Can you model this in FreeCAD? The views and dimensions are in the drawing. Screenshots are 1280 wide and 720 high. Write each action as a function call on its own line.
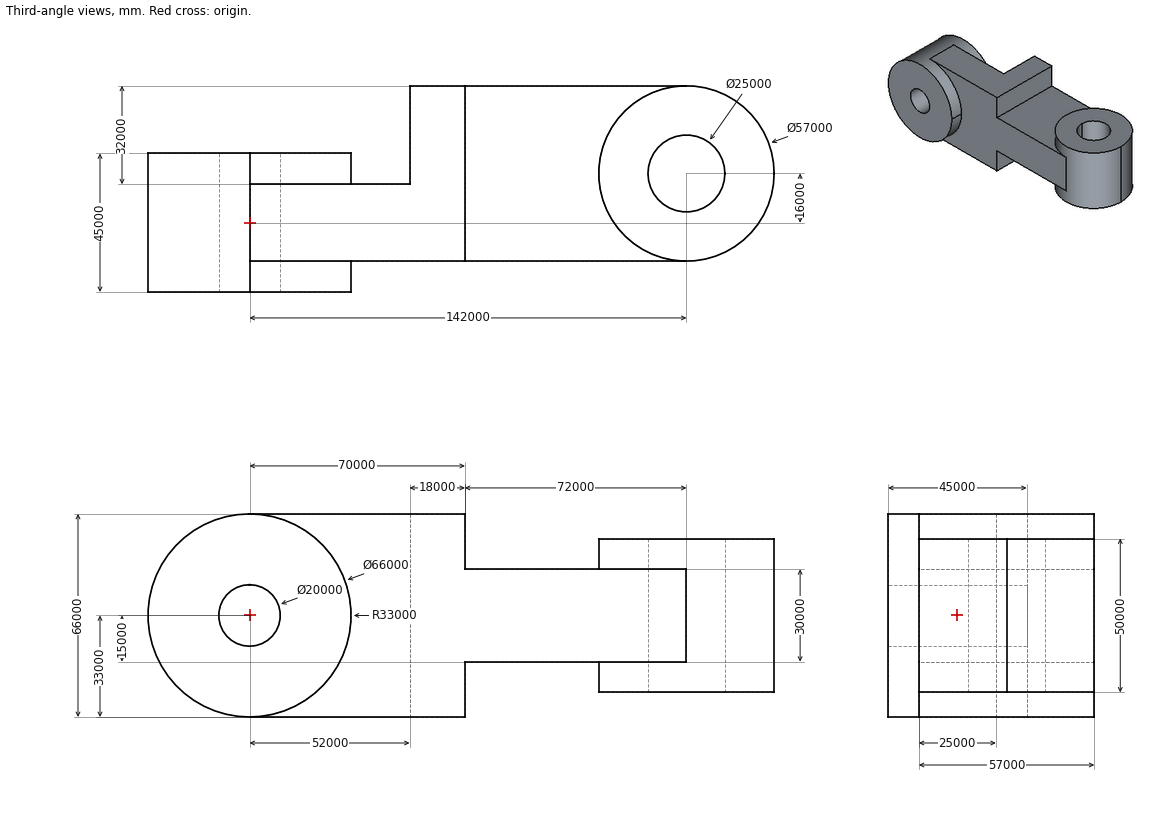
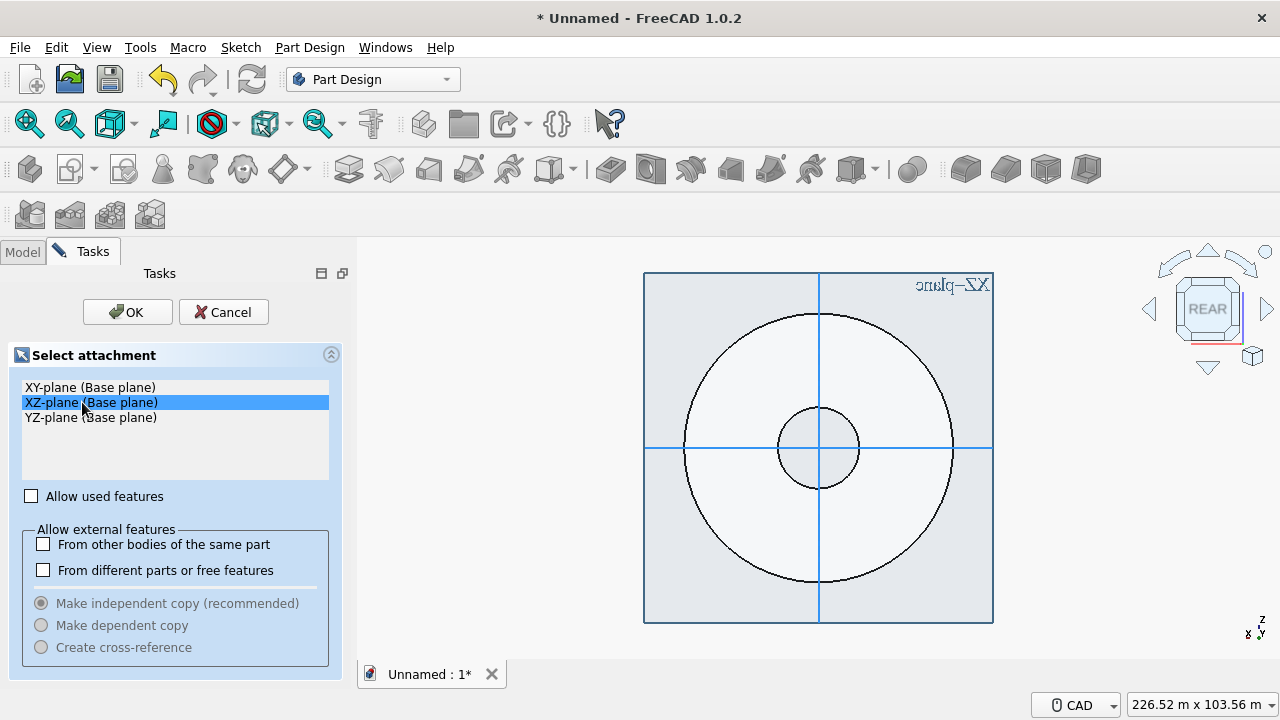
click(128, 312)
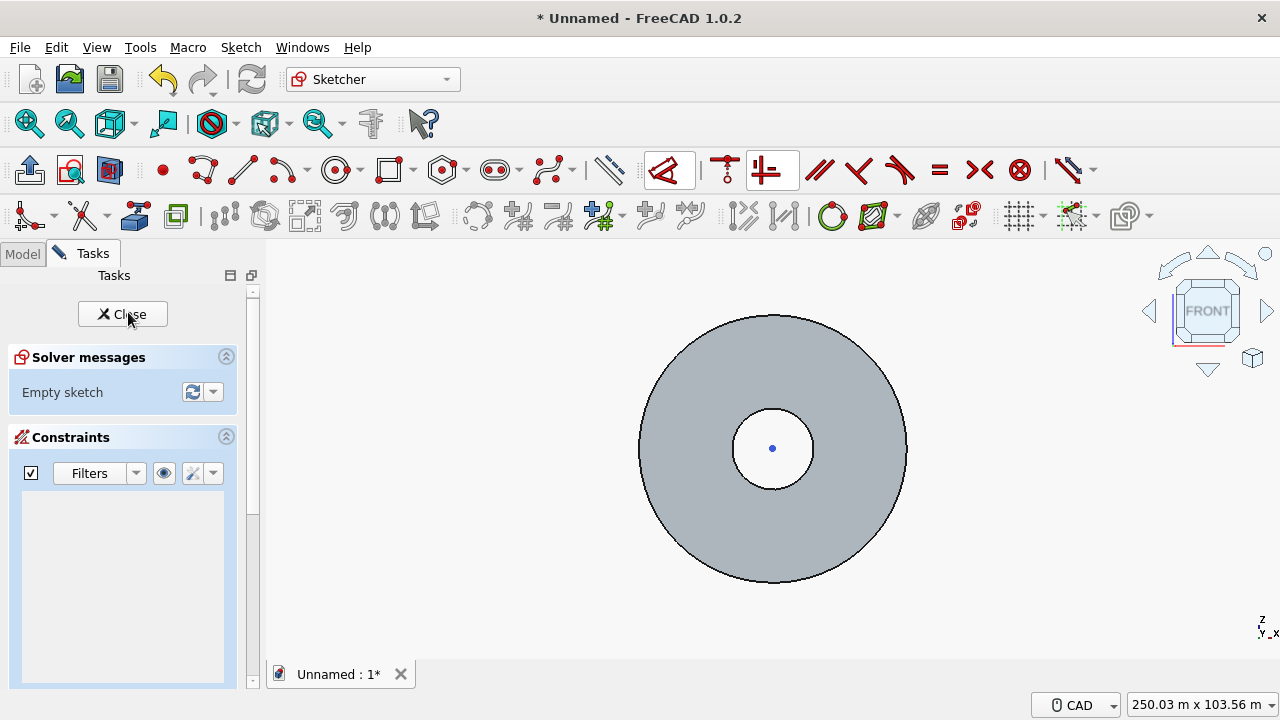
key(q)
key(s)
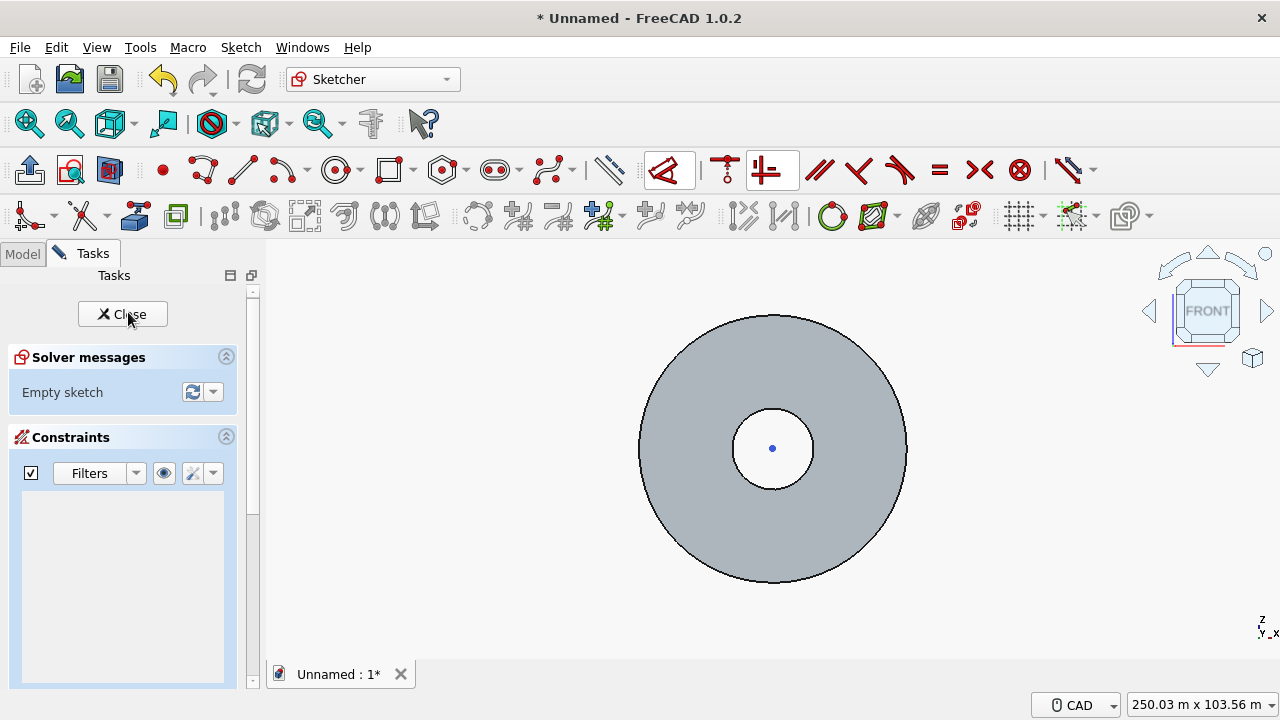
key(g)
key(m)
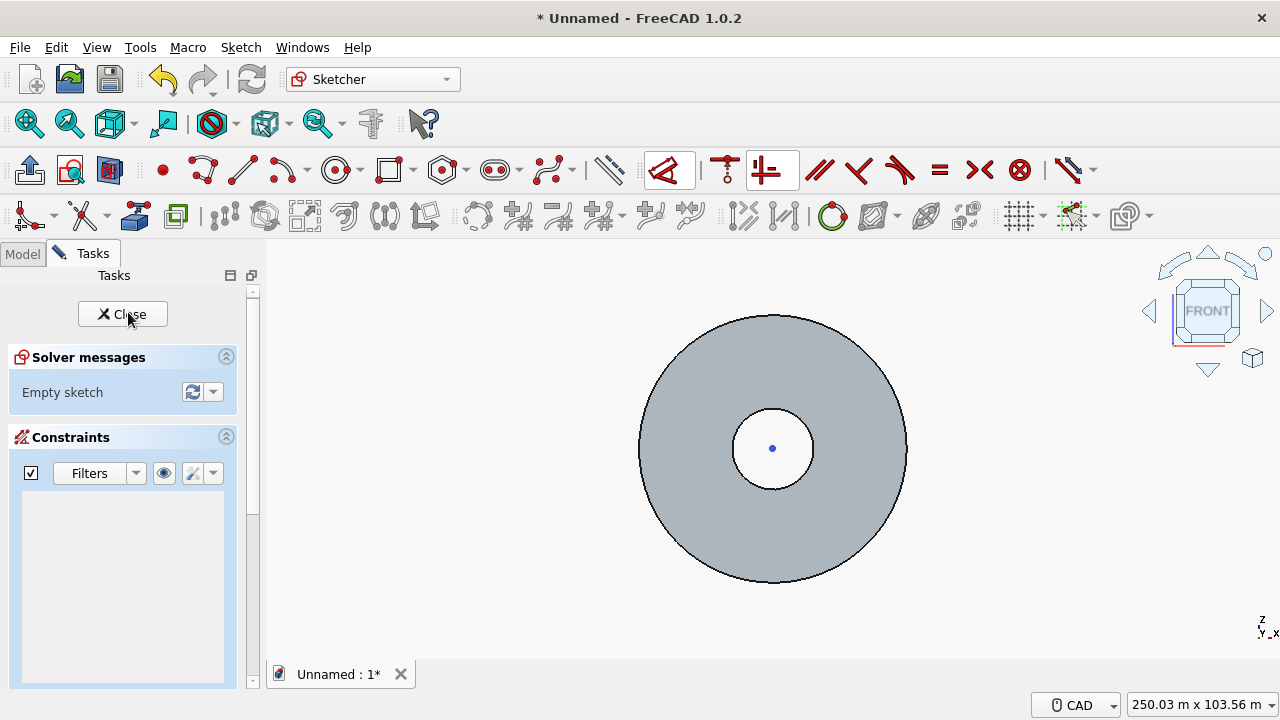
click(773, 315)
click(1057, 315)
click(1057, 583)
click(773, 583)
right_click(773, 583)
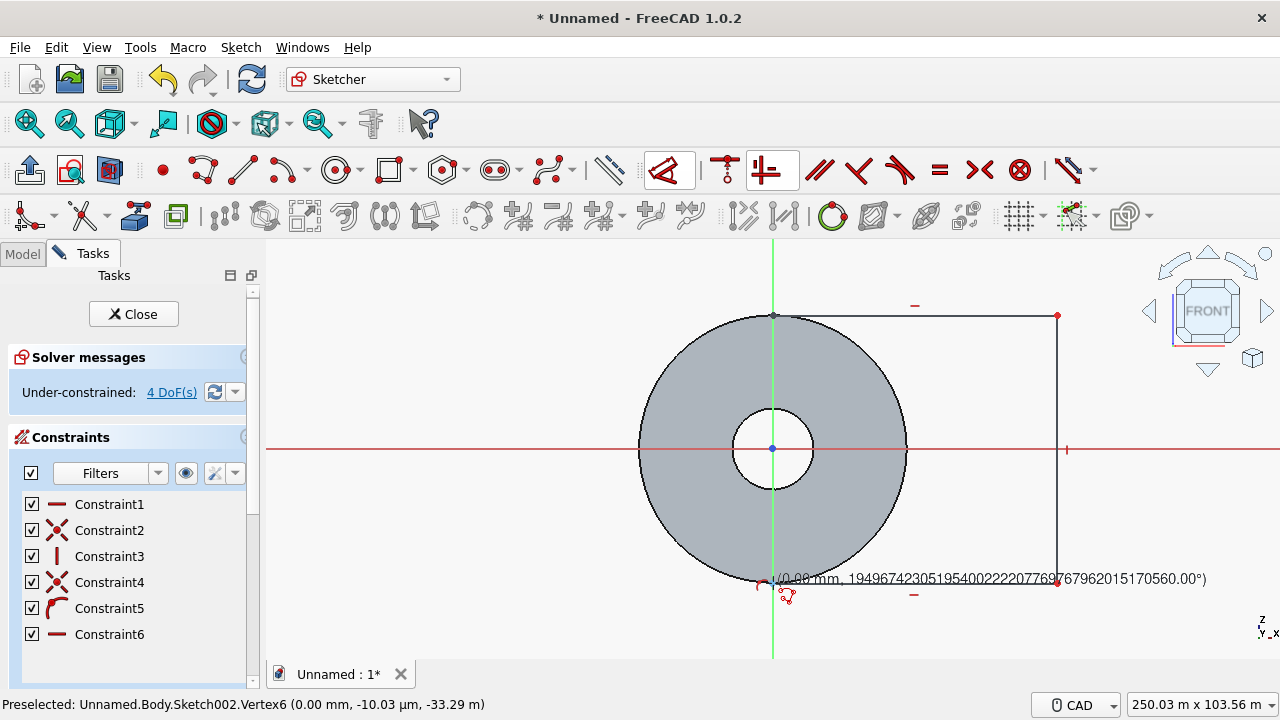
key(g)
key(3)
key(a)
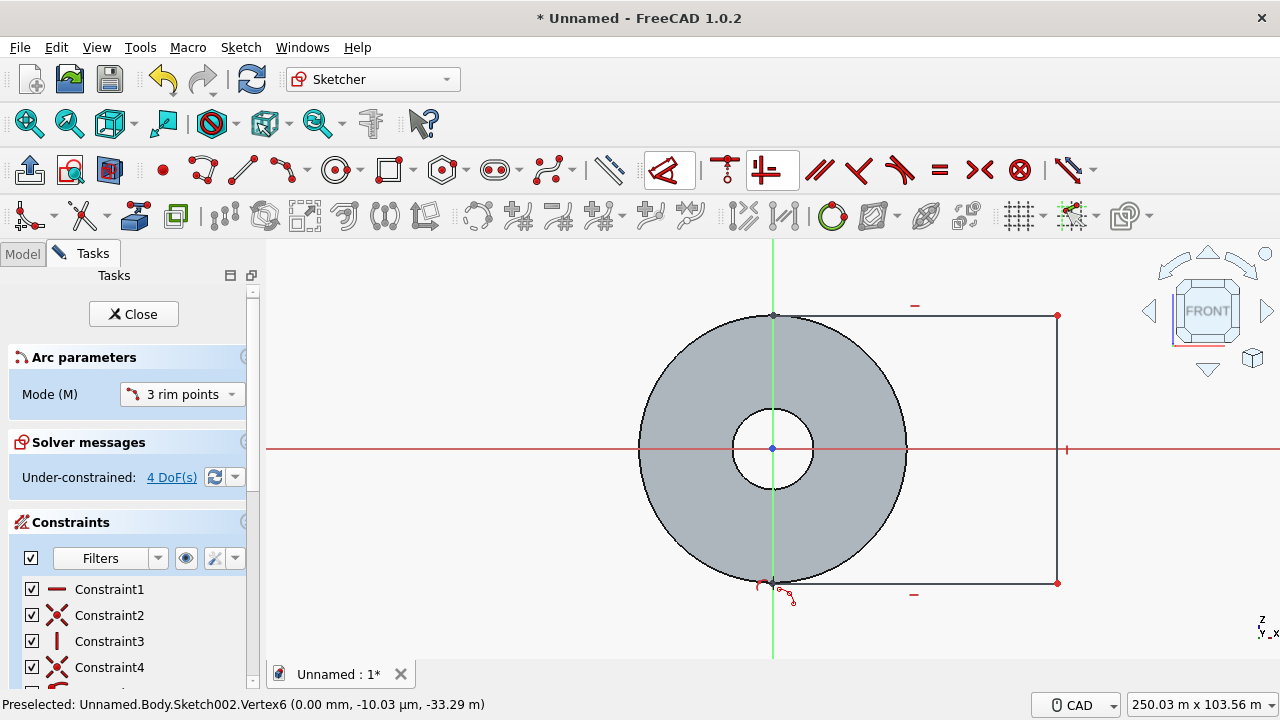
click(773, 584)
click(773, 316)
click(900, 490)
key(Escape)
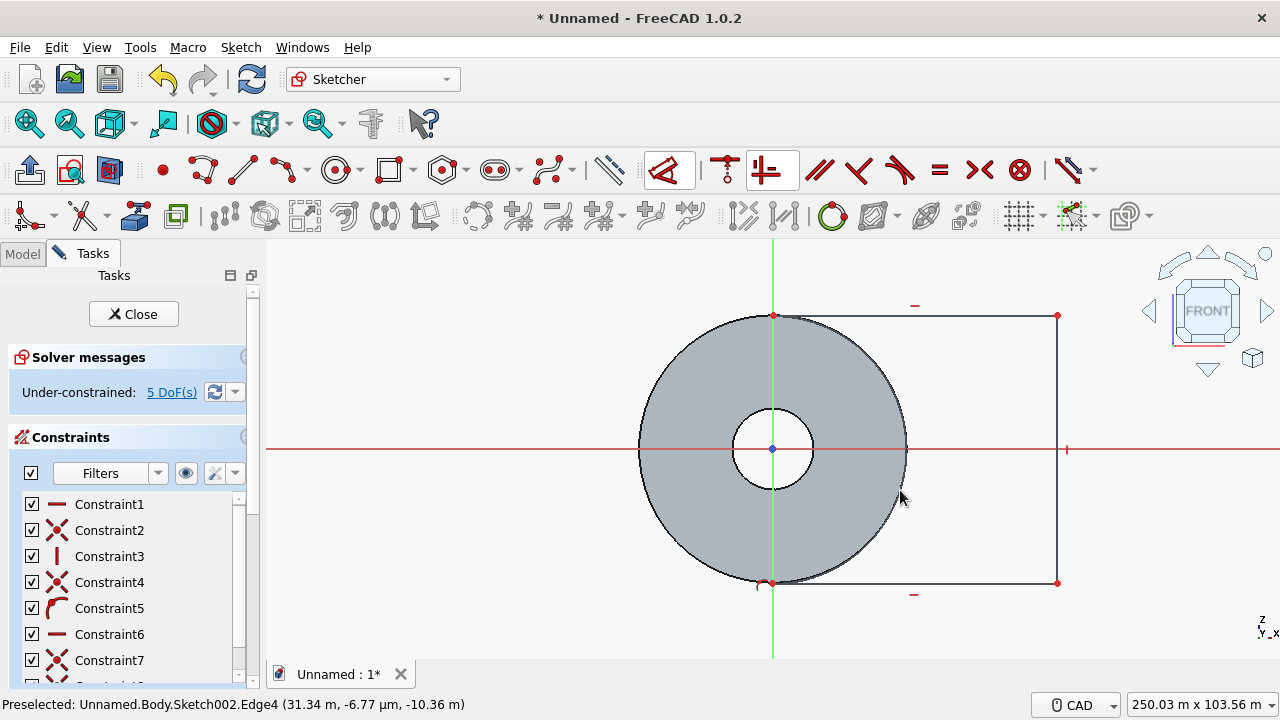
drag(762, 439, 783, 460)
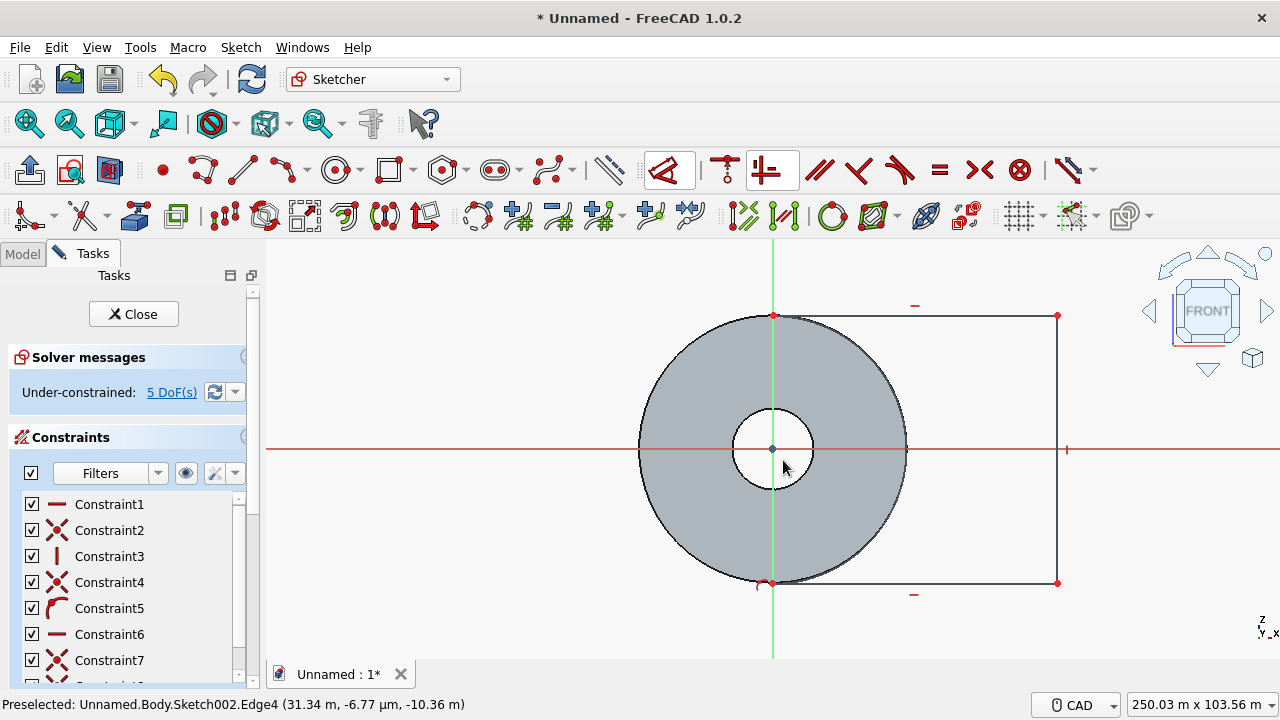
click(726, 170)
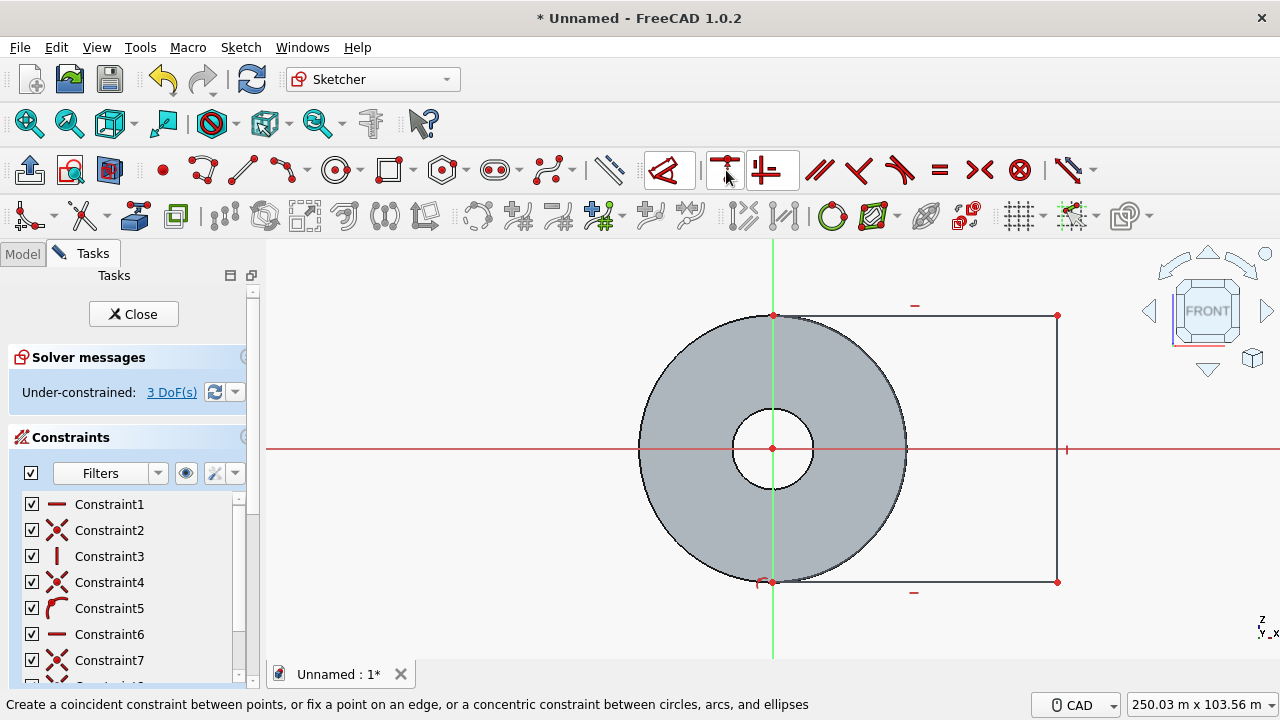
key(d)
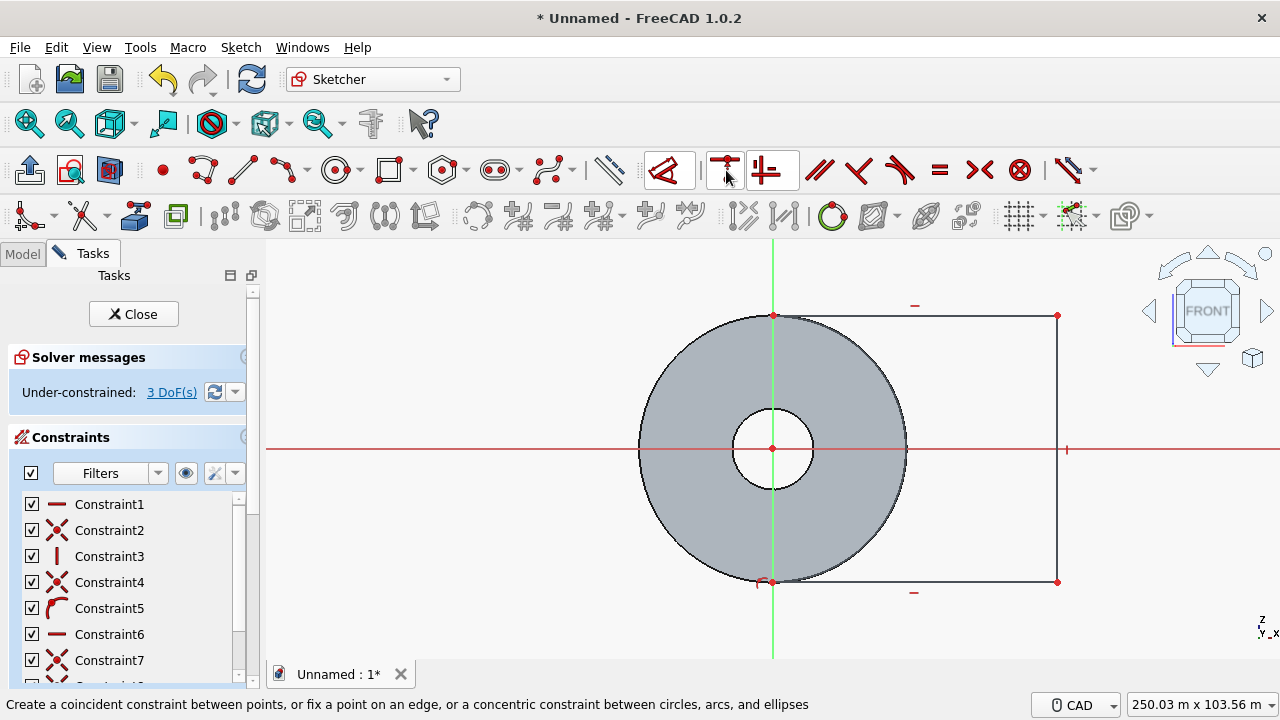
click(880, 527)
click(906, 546)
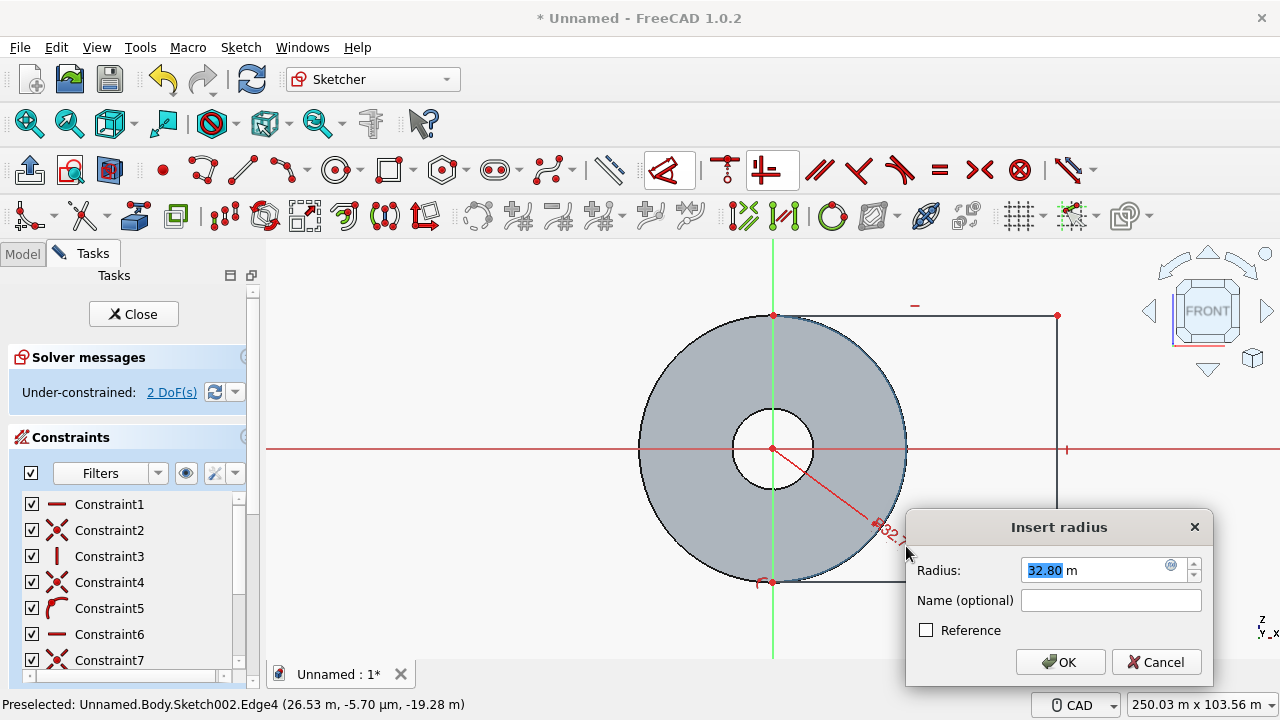
key(ctrl+a)
text(33000 mm)
key(Return)
key(Escape)